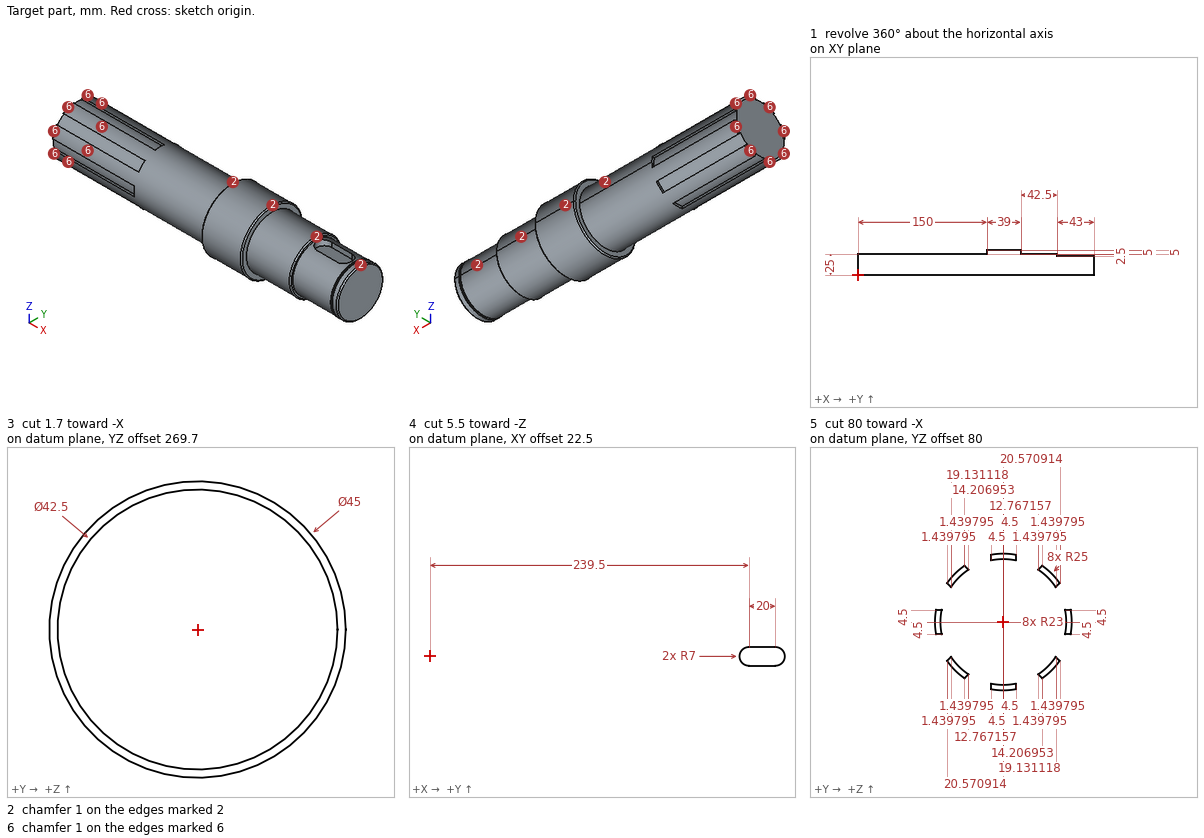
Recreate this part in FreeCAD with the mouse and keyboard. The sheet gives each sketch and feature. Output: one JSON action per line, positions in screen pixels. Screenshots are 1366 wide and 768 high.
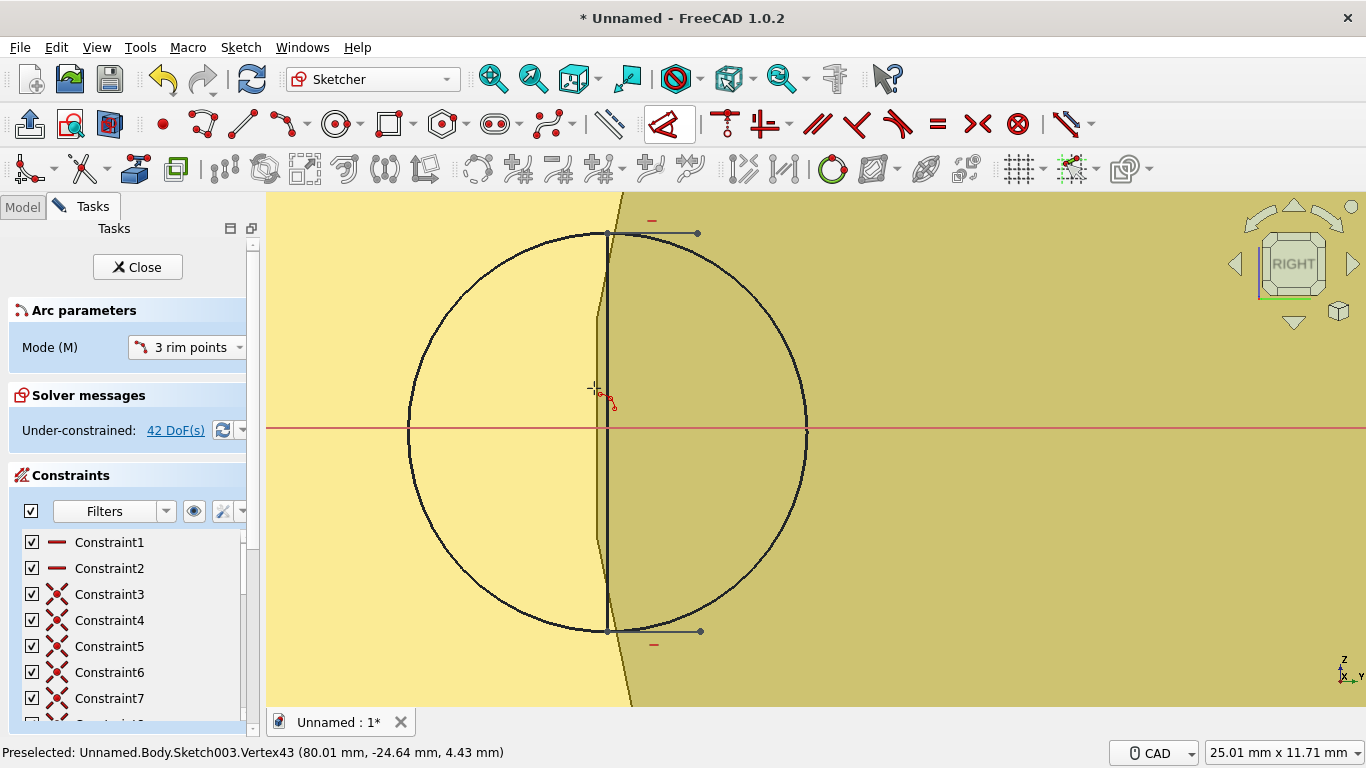
{"action": "left_click", "coordinate": [592, 388]}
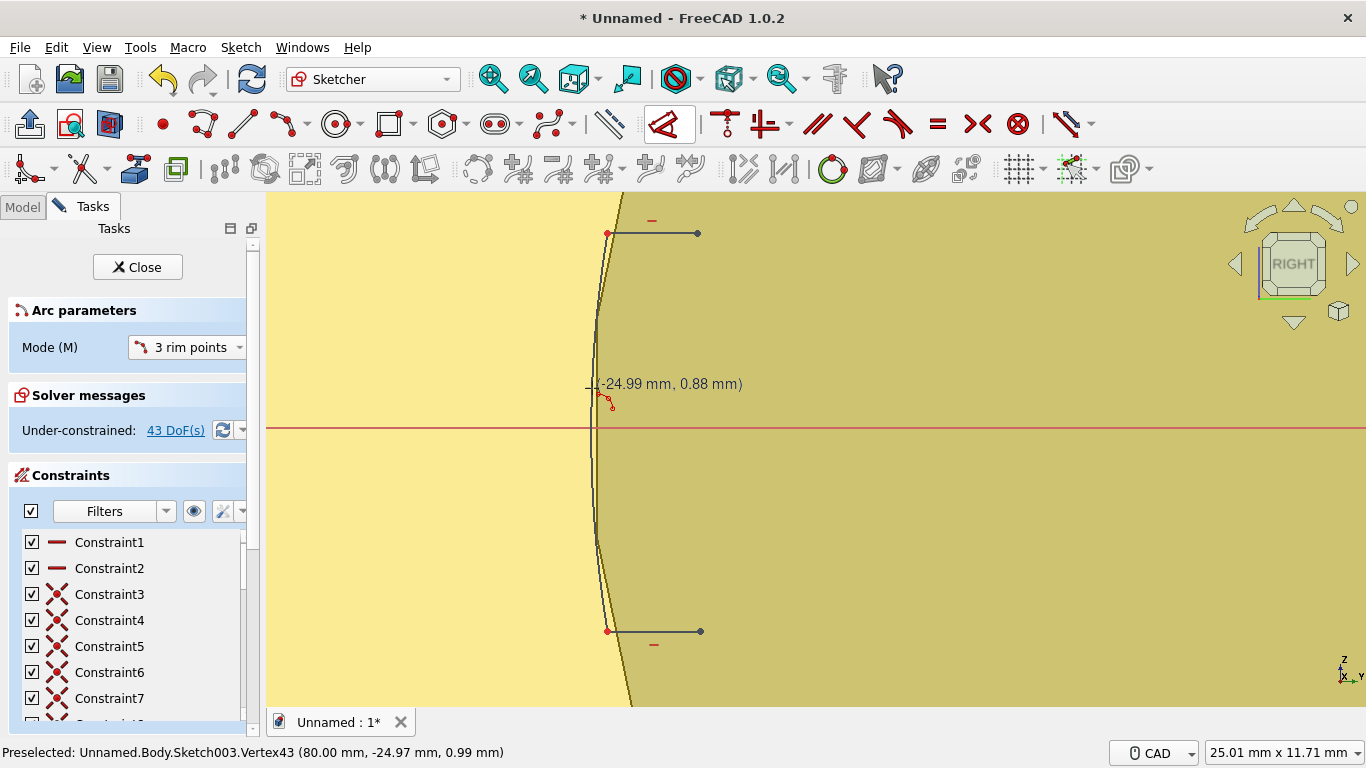
{"action": "left_click", "coordinate": [697, 233]}
{"action": "left_click", "coordinate": [701, 632]}
{"action": "left_click", "coordinate": [681, 388]}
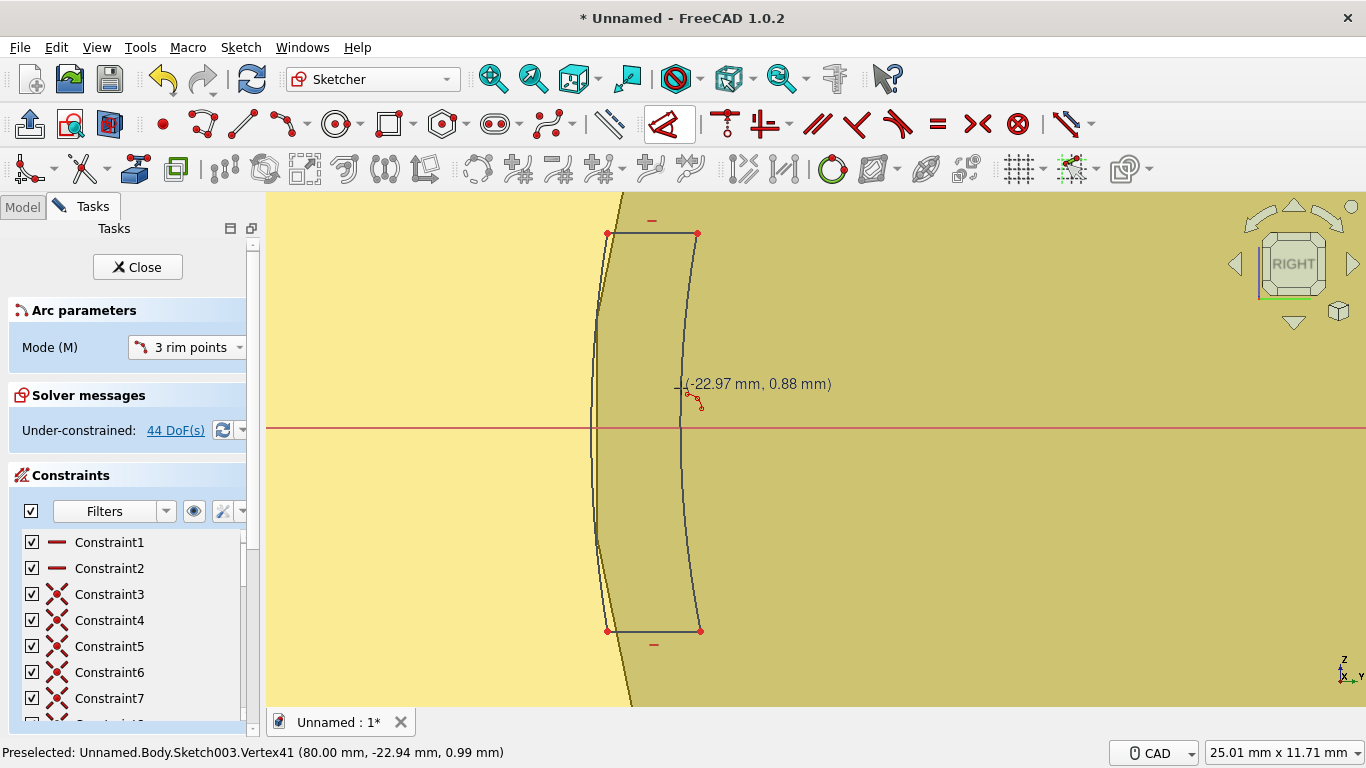
{"action": "left_click", "coordinate": [244, 124]}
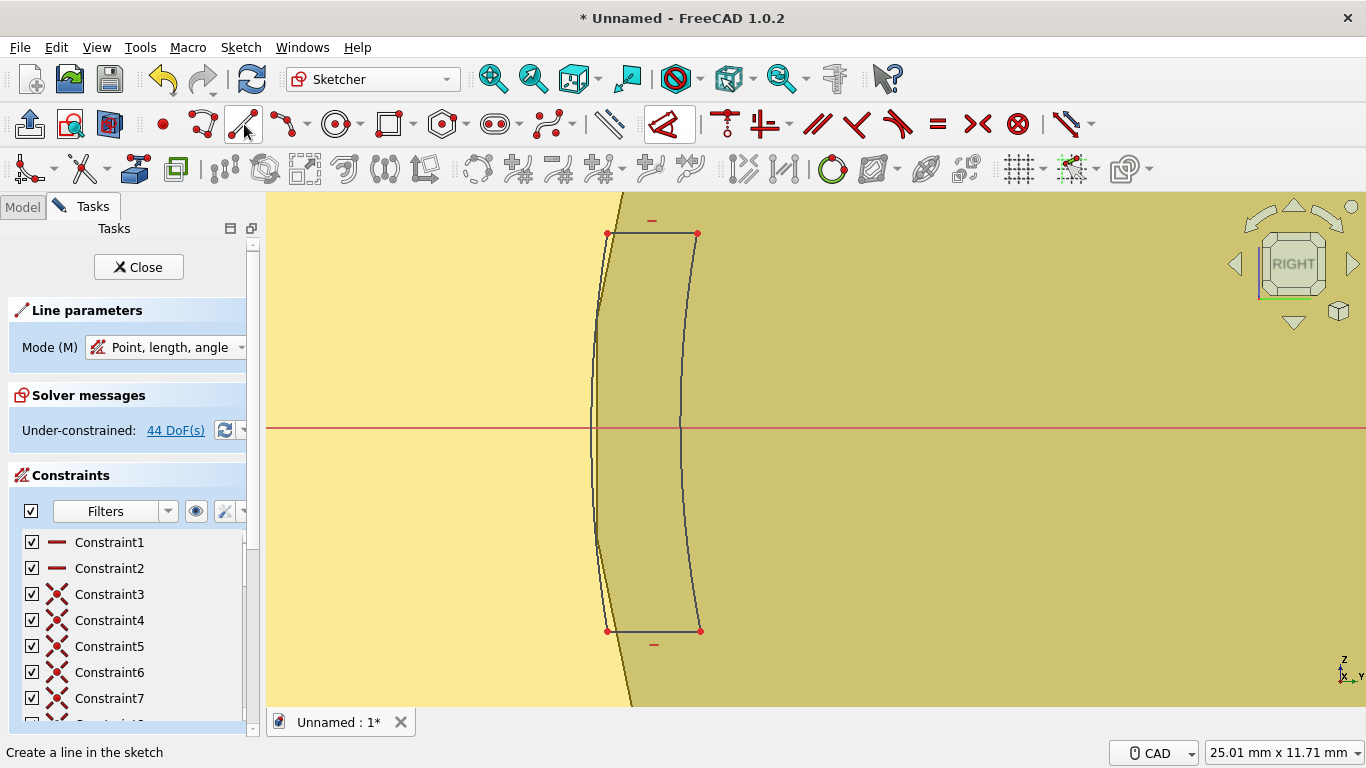
{"action": "scroll", "coordinate": [600, 453], "scroll_direction": "down", "scroll_amount": 10}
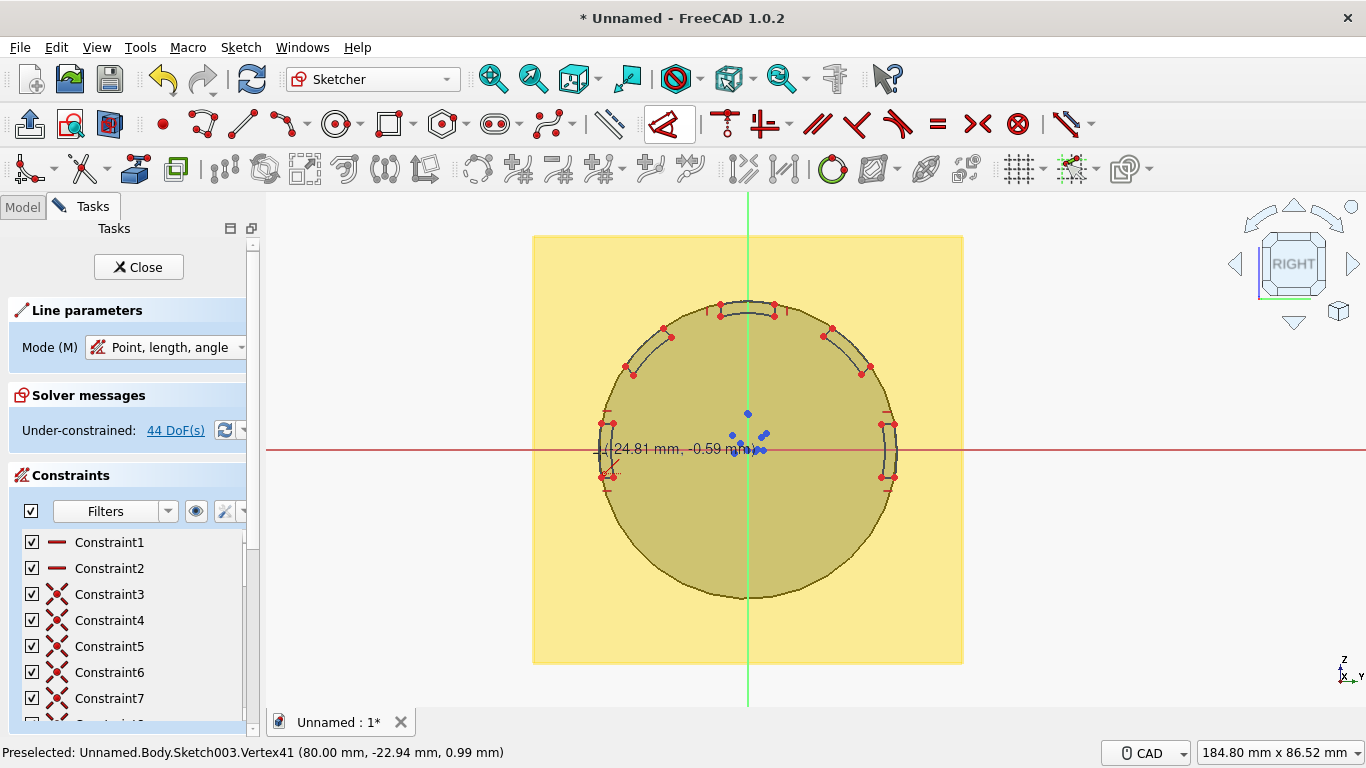
{"action": "left_click", "coordinate": [672, 564]}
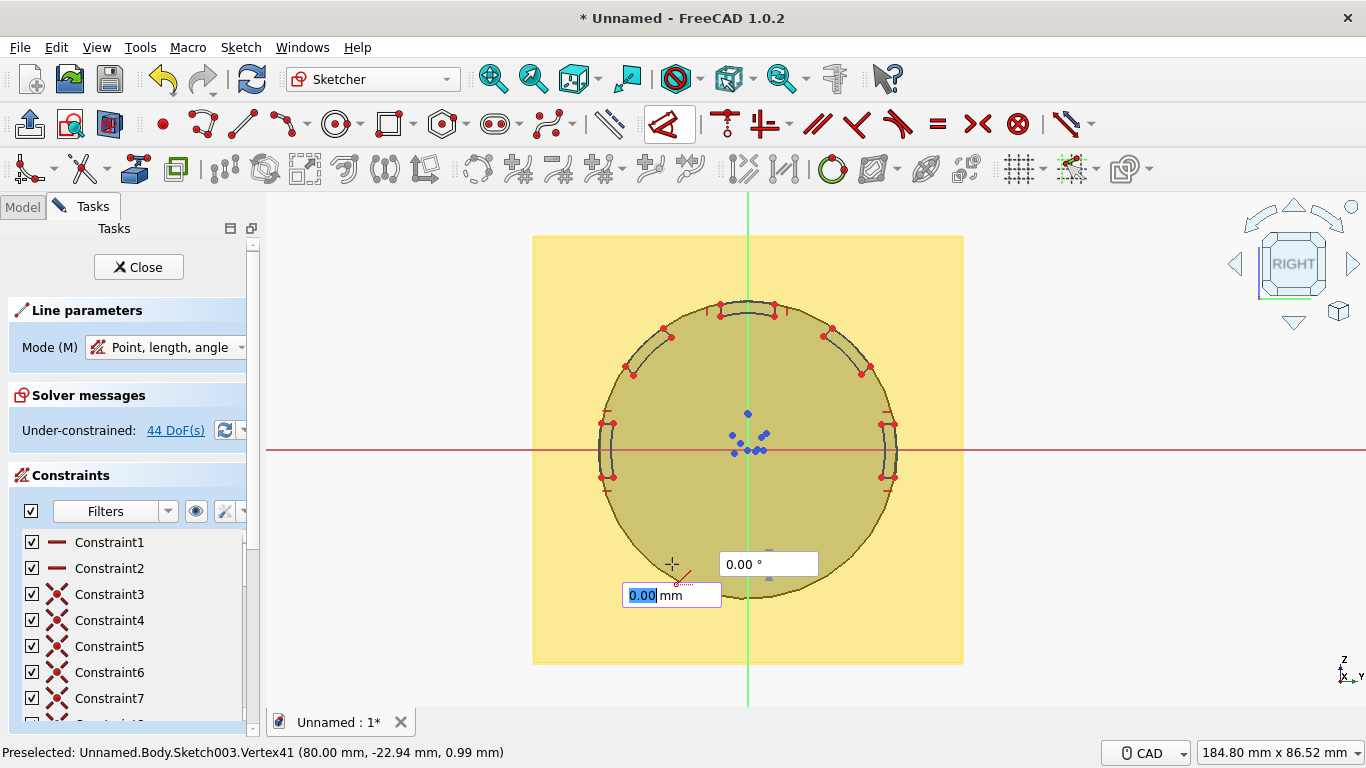
{"action": "scroll", "coordinate": [663, 572], "scroll_direction": "up", "scroll_amount": 2}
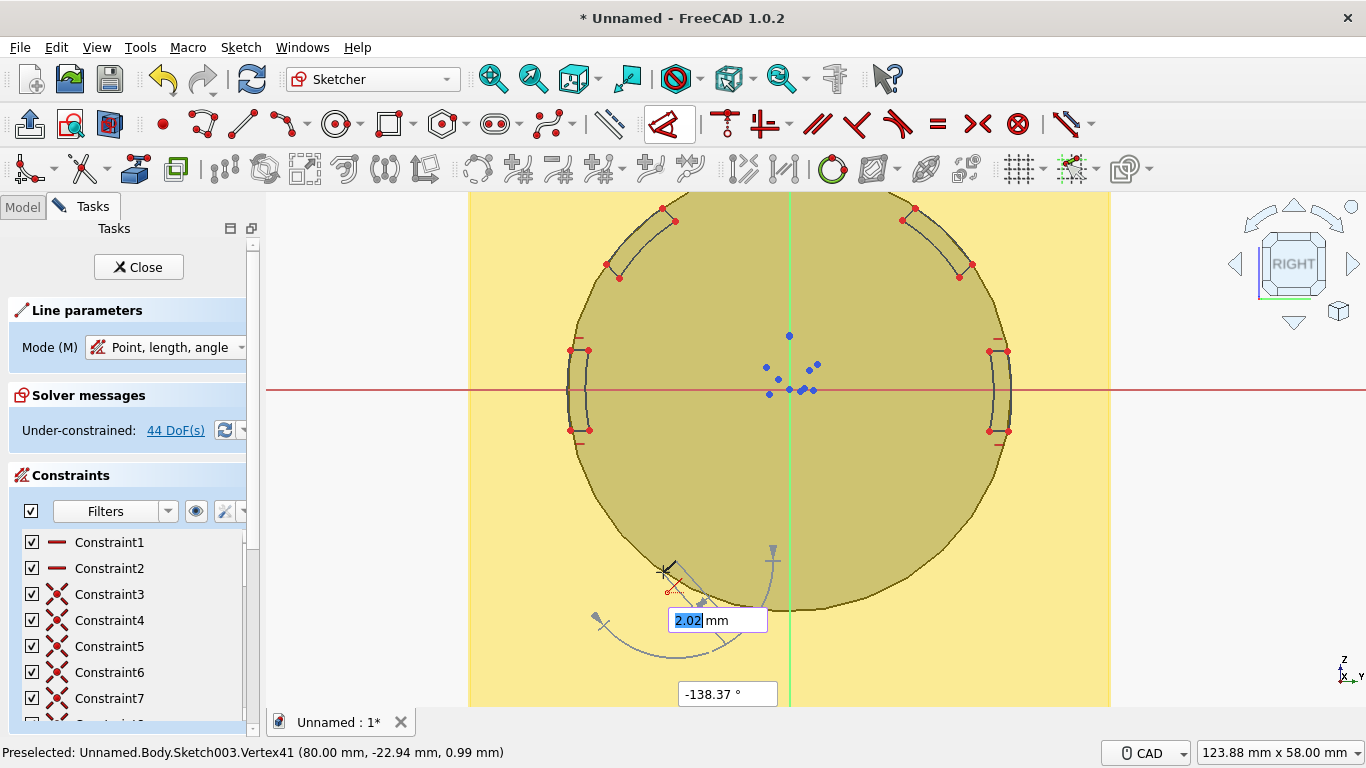
{"action": "left_click", "coordinate": [663, 572]}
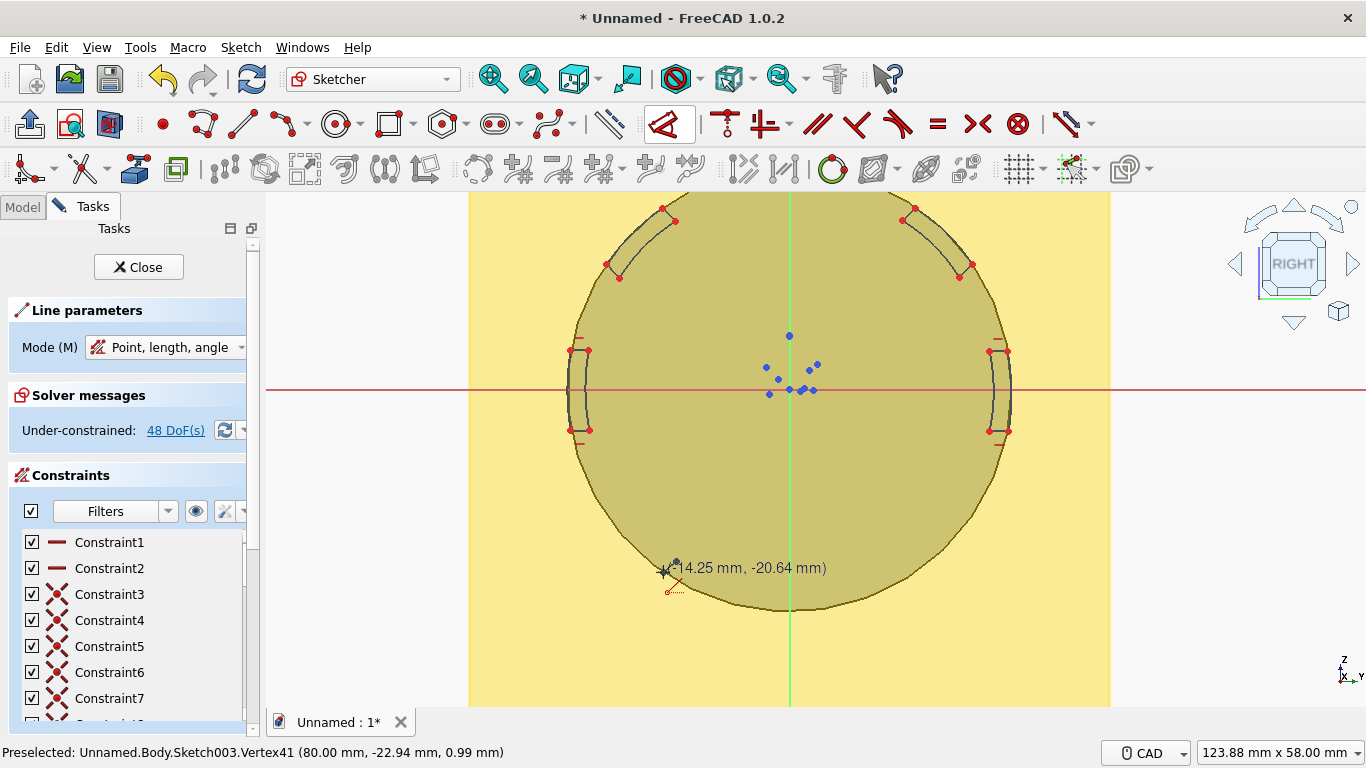
{"action": "left_click", "coordinate": [607, 516]}
{"action": "left_click", "coordinate": [620, 503]}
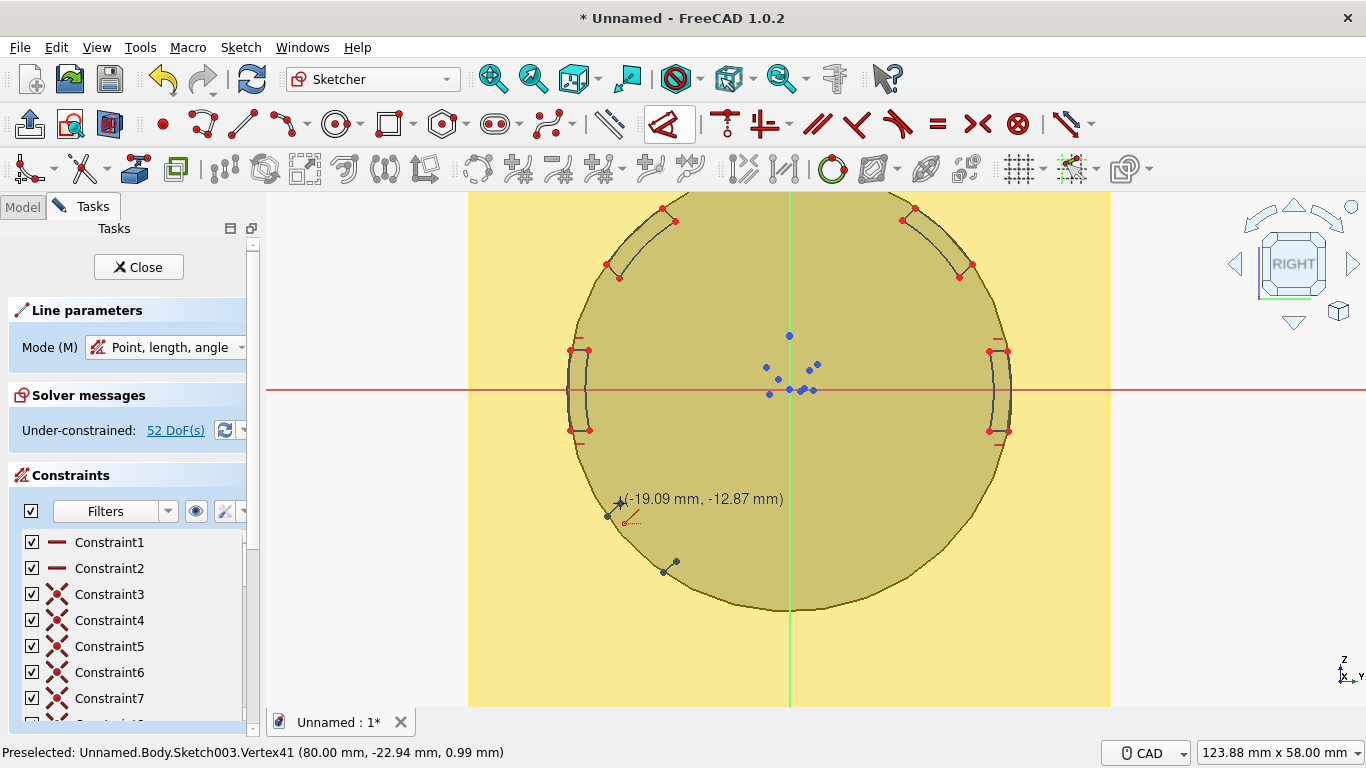
{"action": "left_click", "coordinate": [284, 124]}